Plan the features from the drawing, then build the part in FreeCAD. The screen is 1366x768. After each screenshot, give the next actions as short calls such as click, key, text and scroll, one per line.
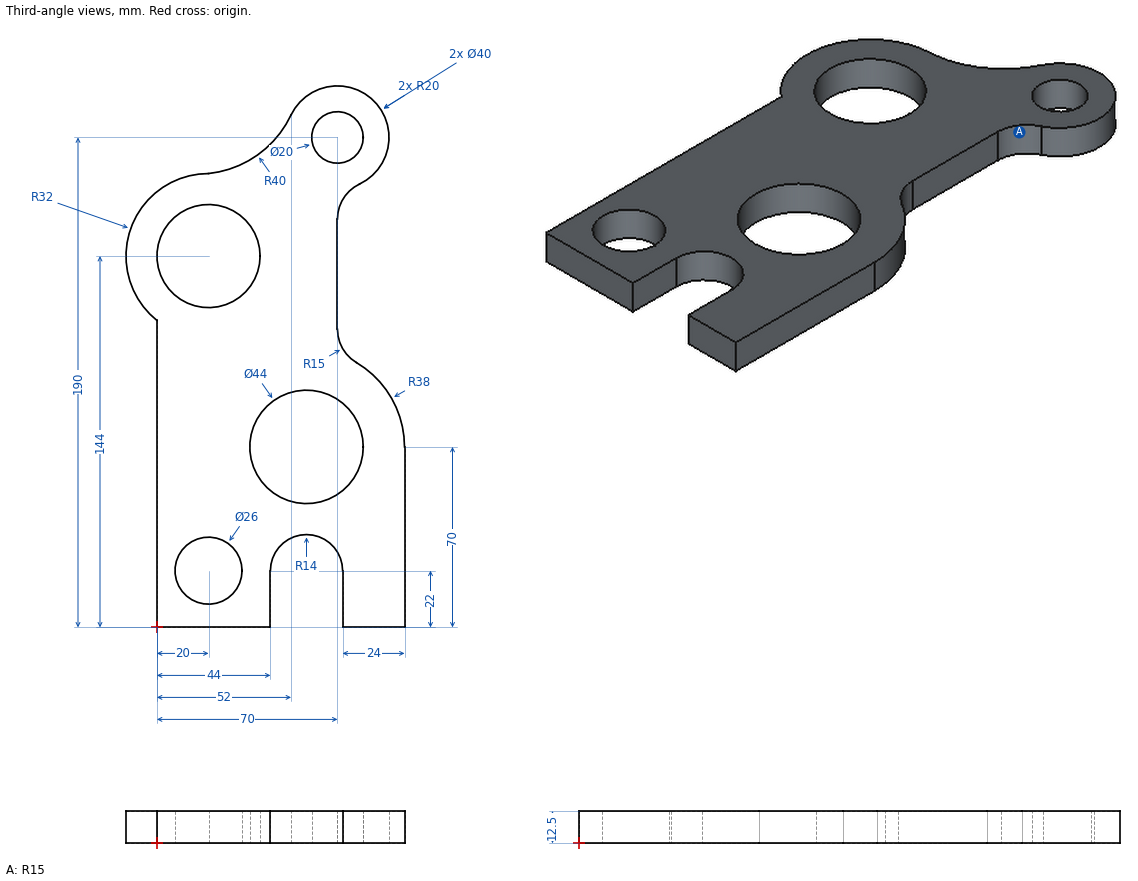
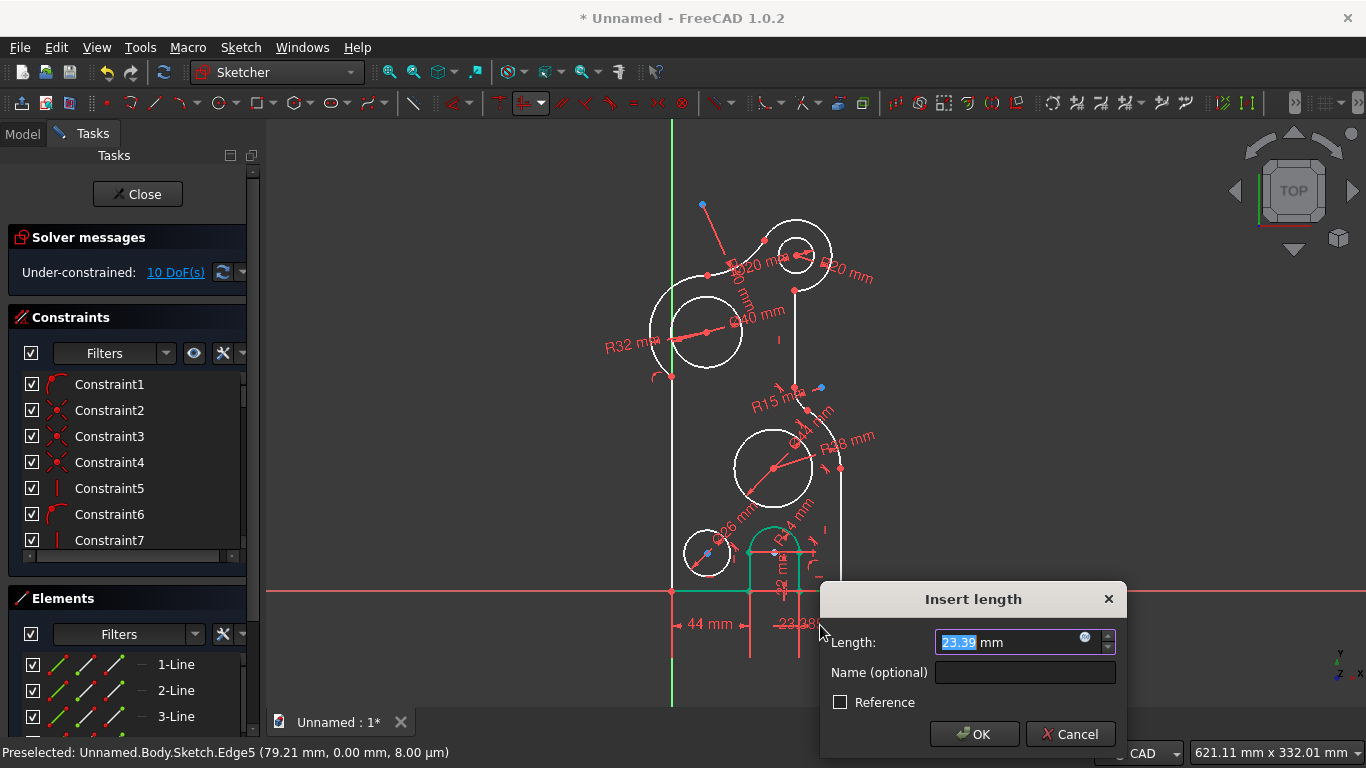
text(24)
key(Return)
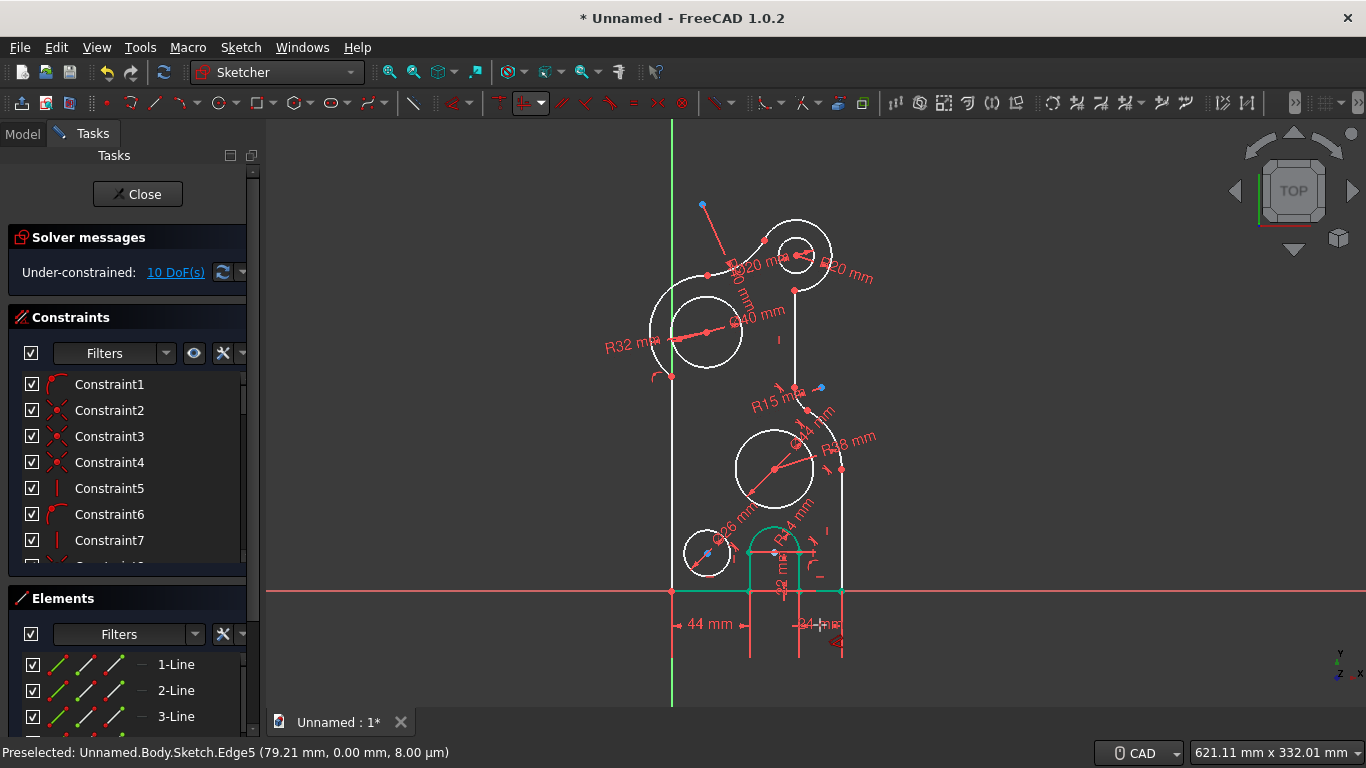
click(842, 554)
click(876, 530)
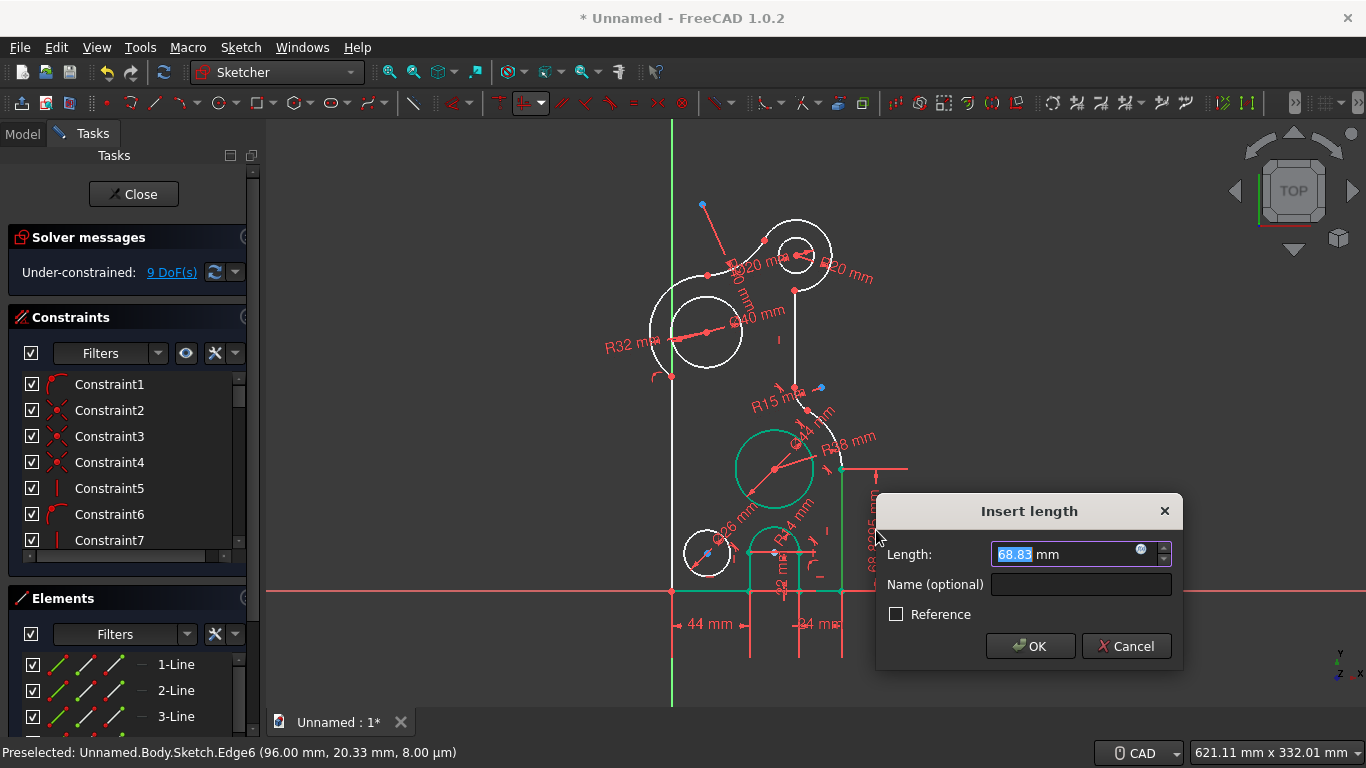
text(70)
key(Return)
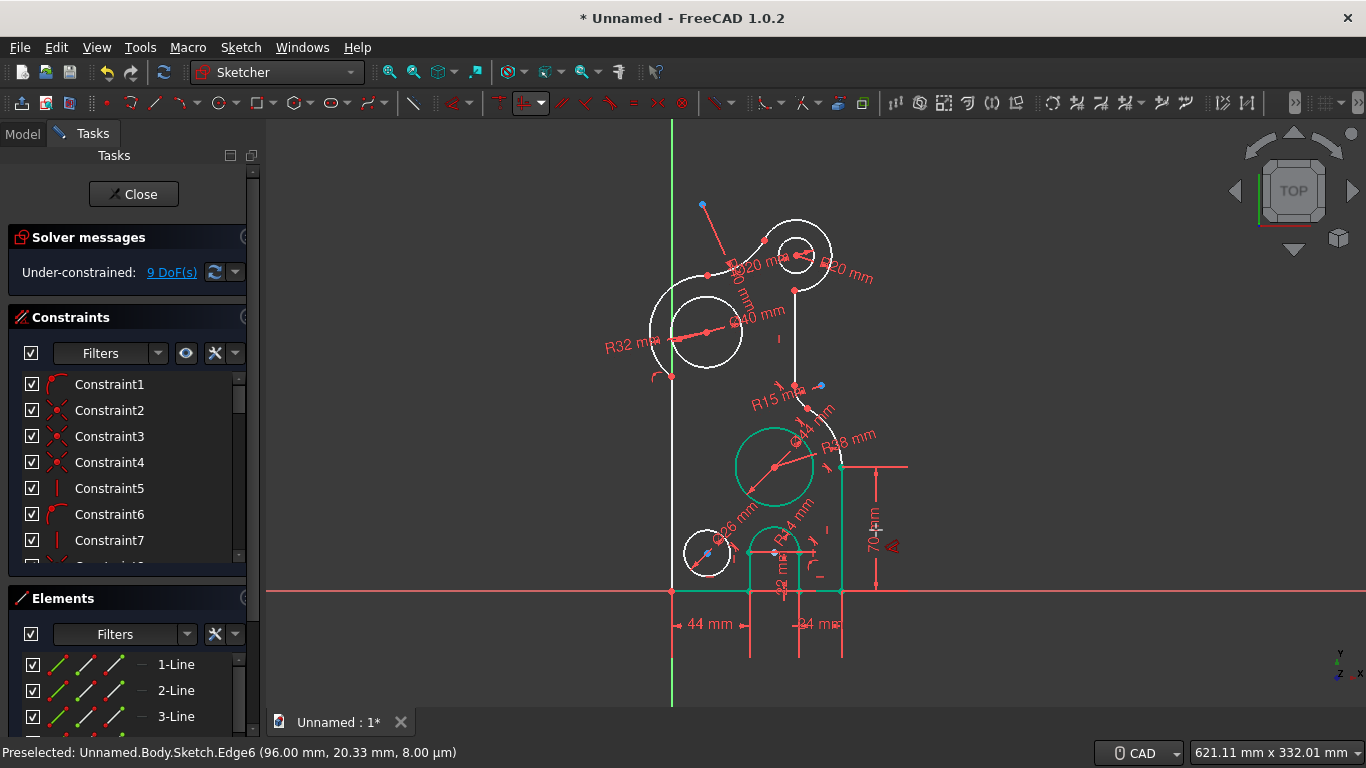
click(707, 553)
click(689, 649)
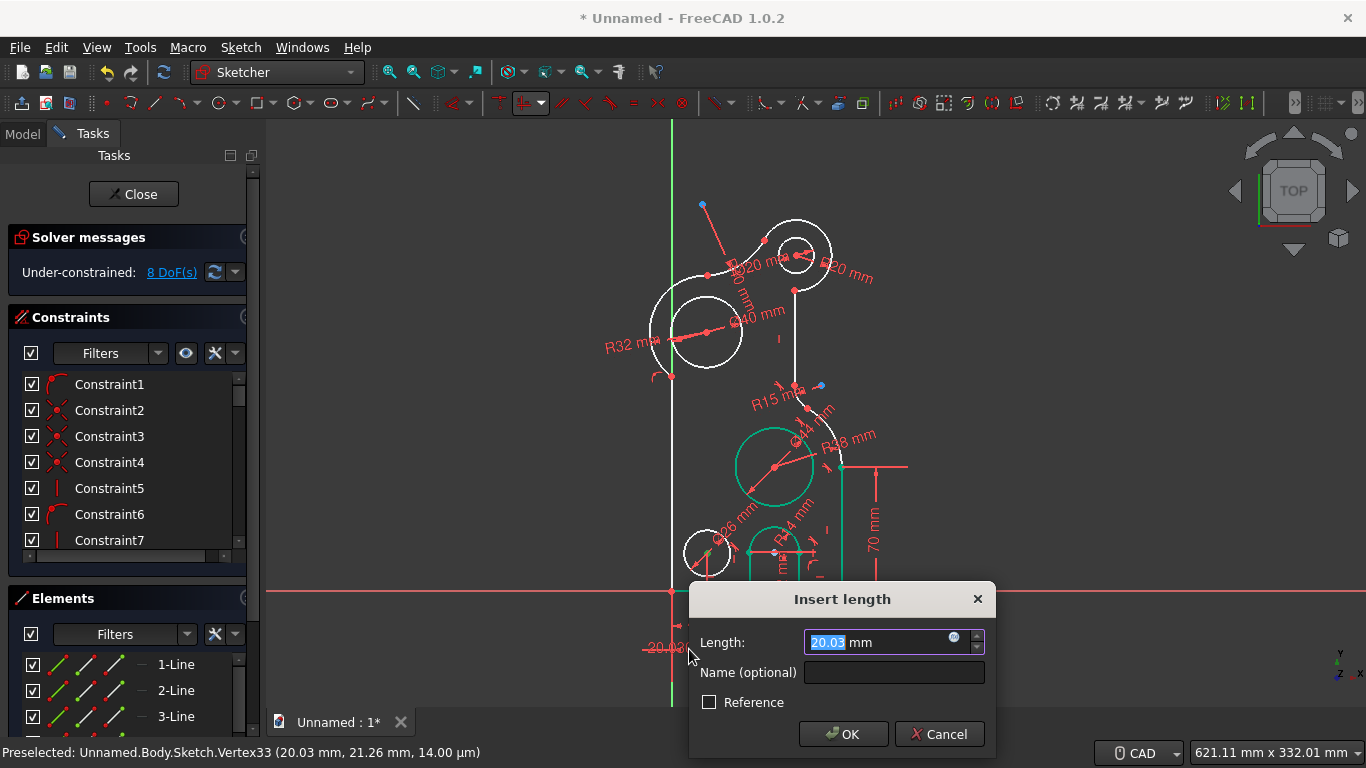
text(20)
key(Return)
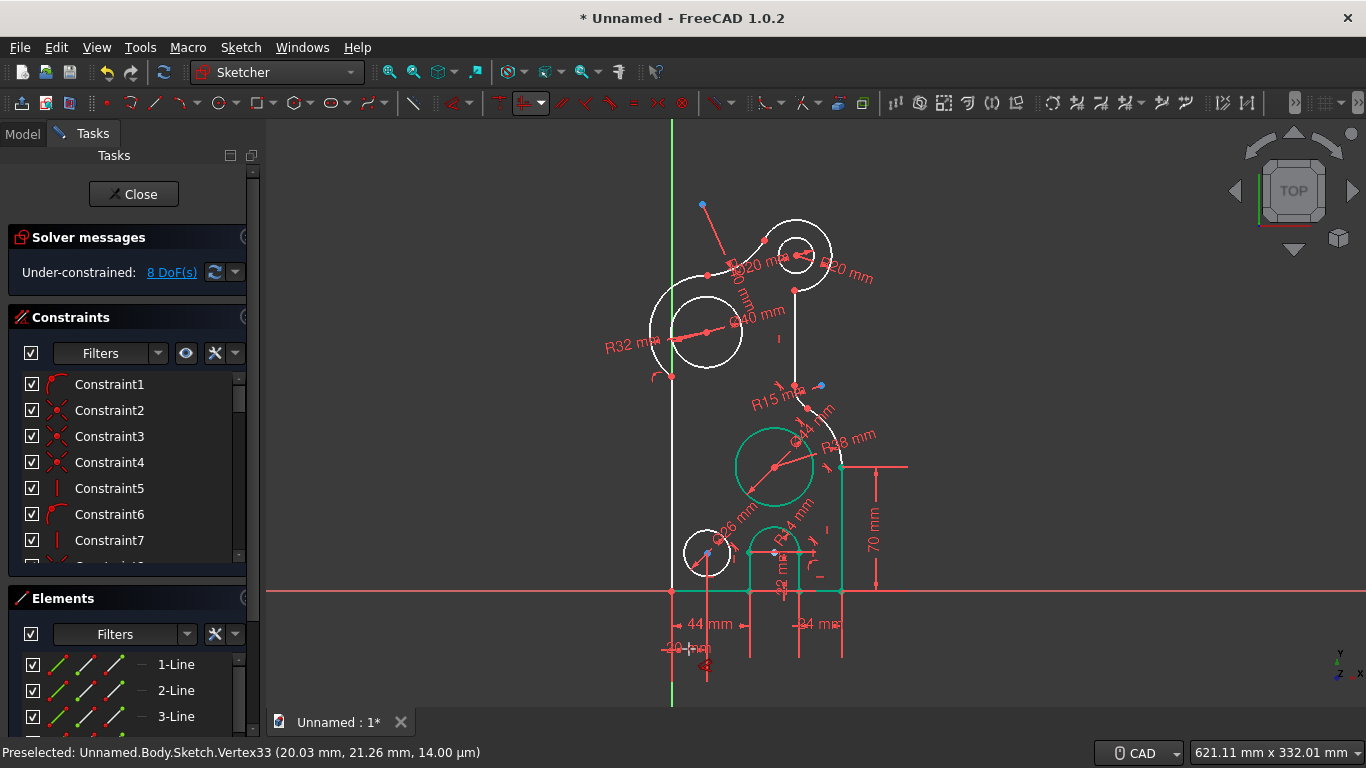
click(707, 553)
click(638, 572)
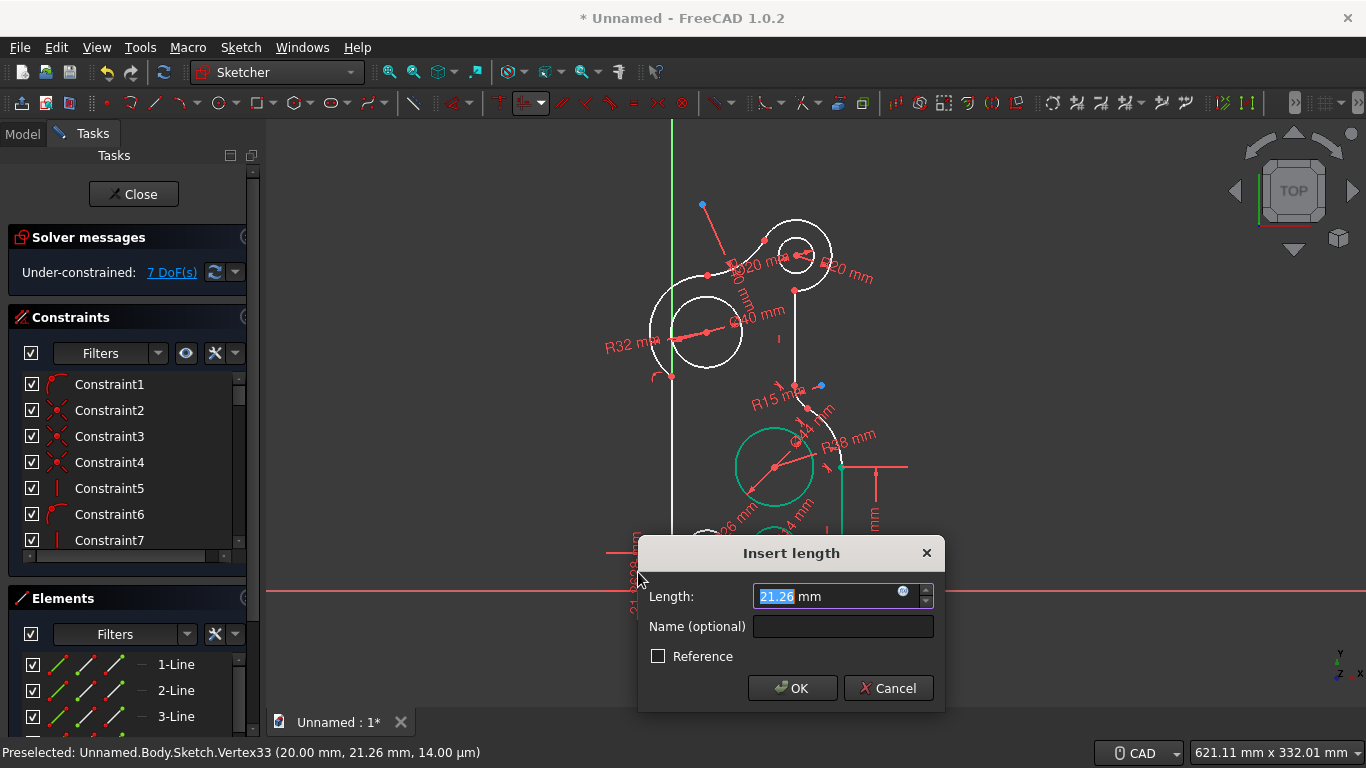
text(22)
key(Return)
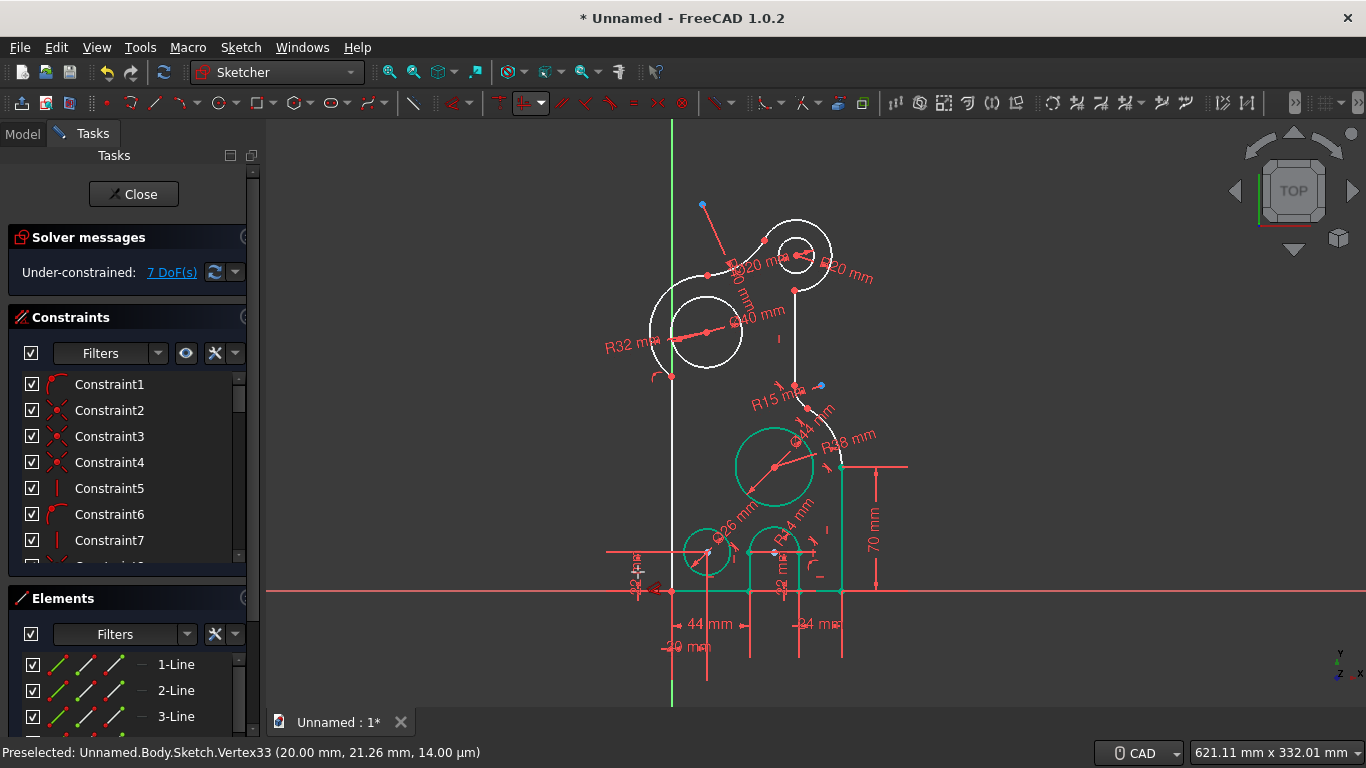
click(706, 332)
click(689, 673)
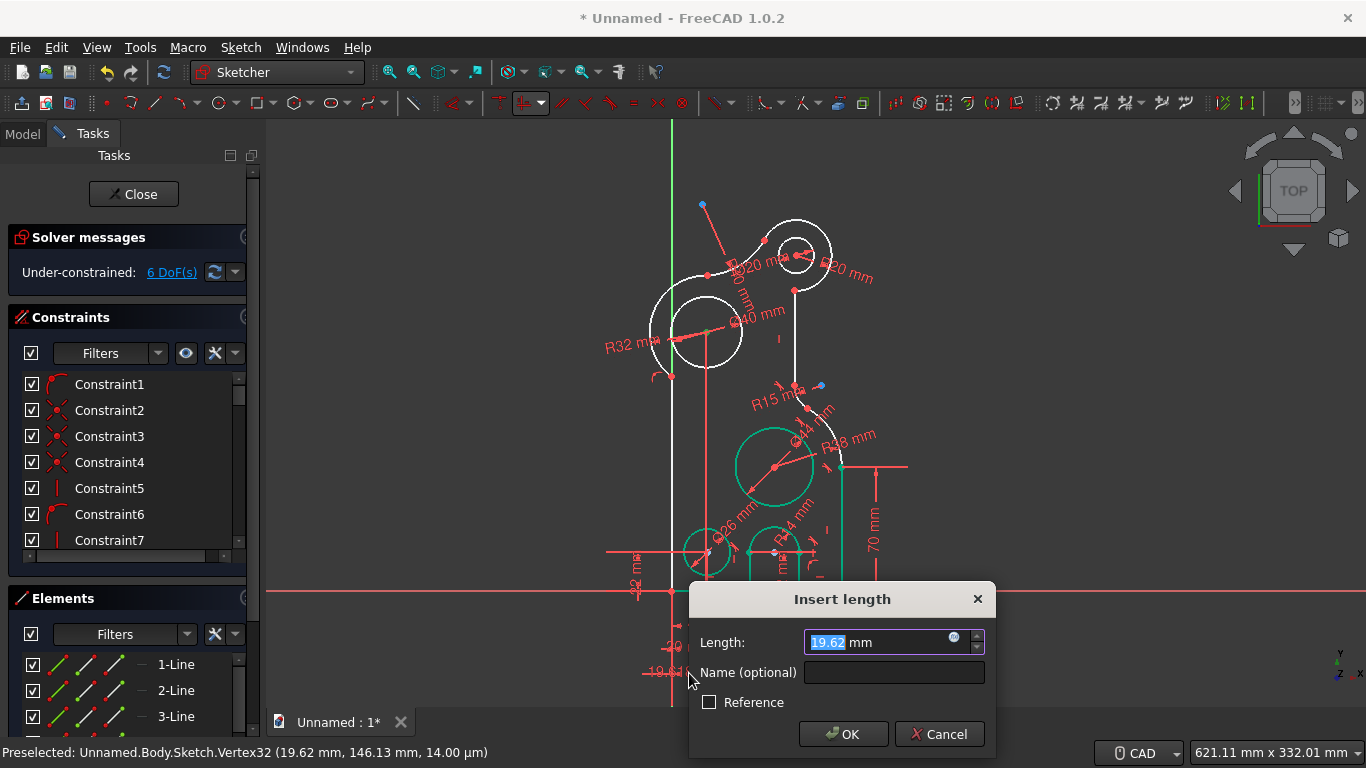
text(20)
key(Return)